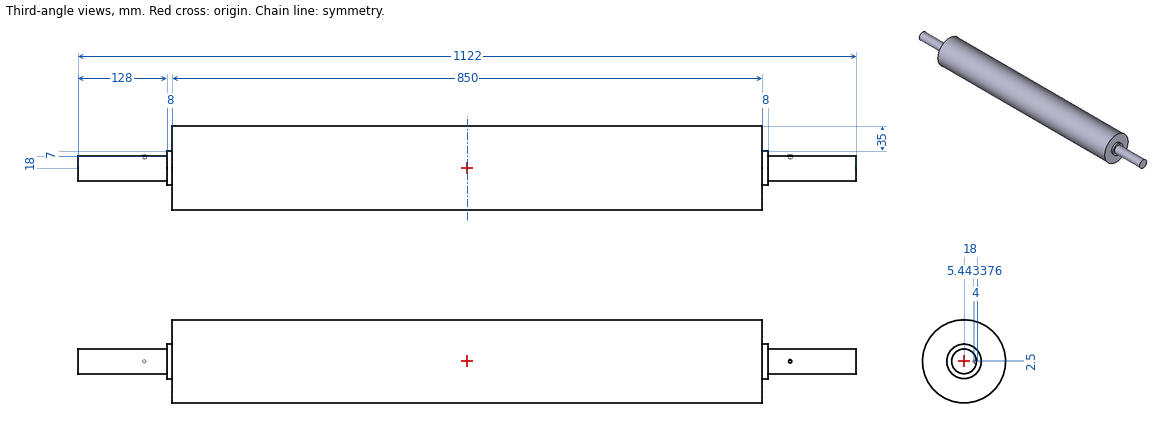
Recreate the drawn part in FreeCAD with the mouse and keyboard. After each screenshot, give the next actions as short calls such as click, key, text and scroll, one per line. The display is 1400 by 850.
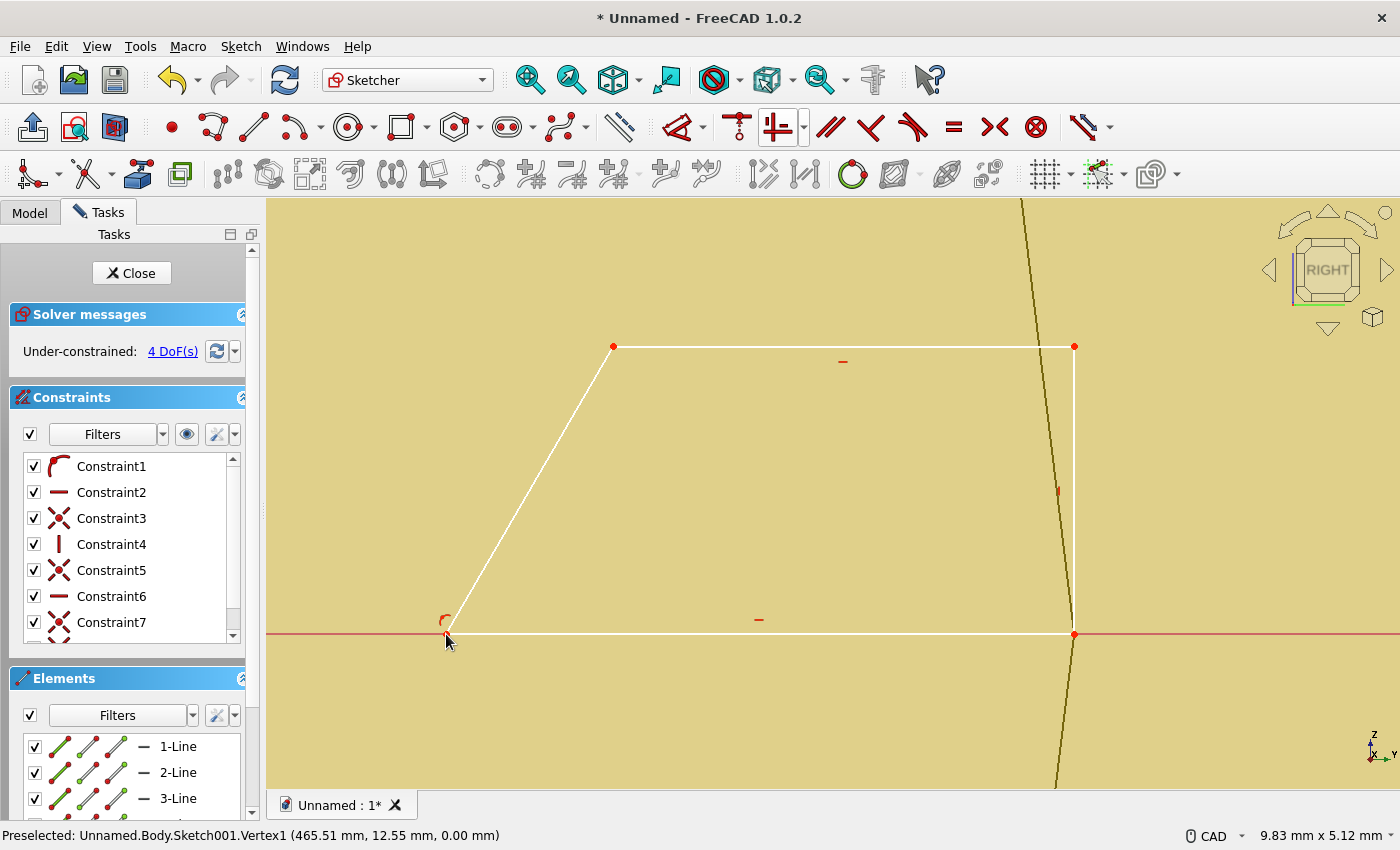
click(676, 128)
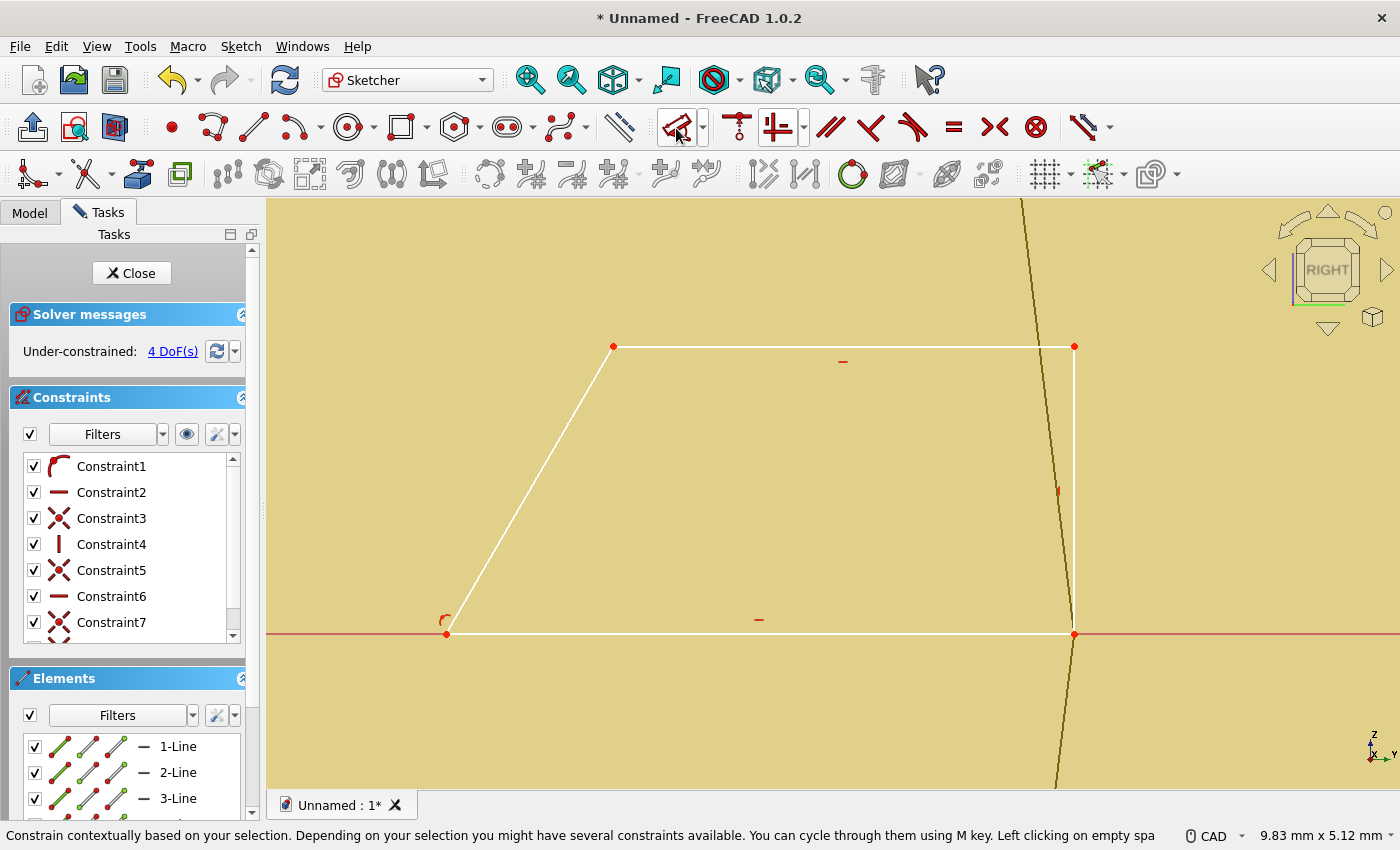
click(936, 347)
click(844, 313)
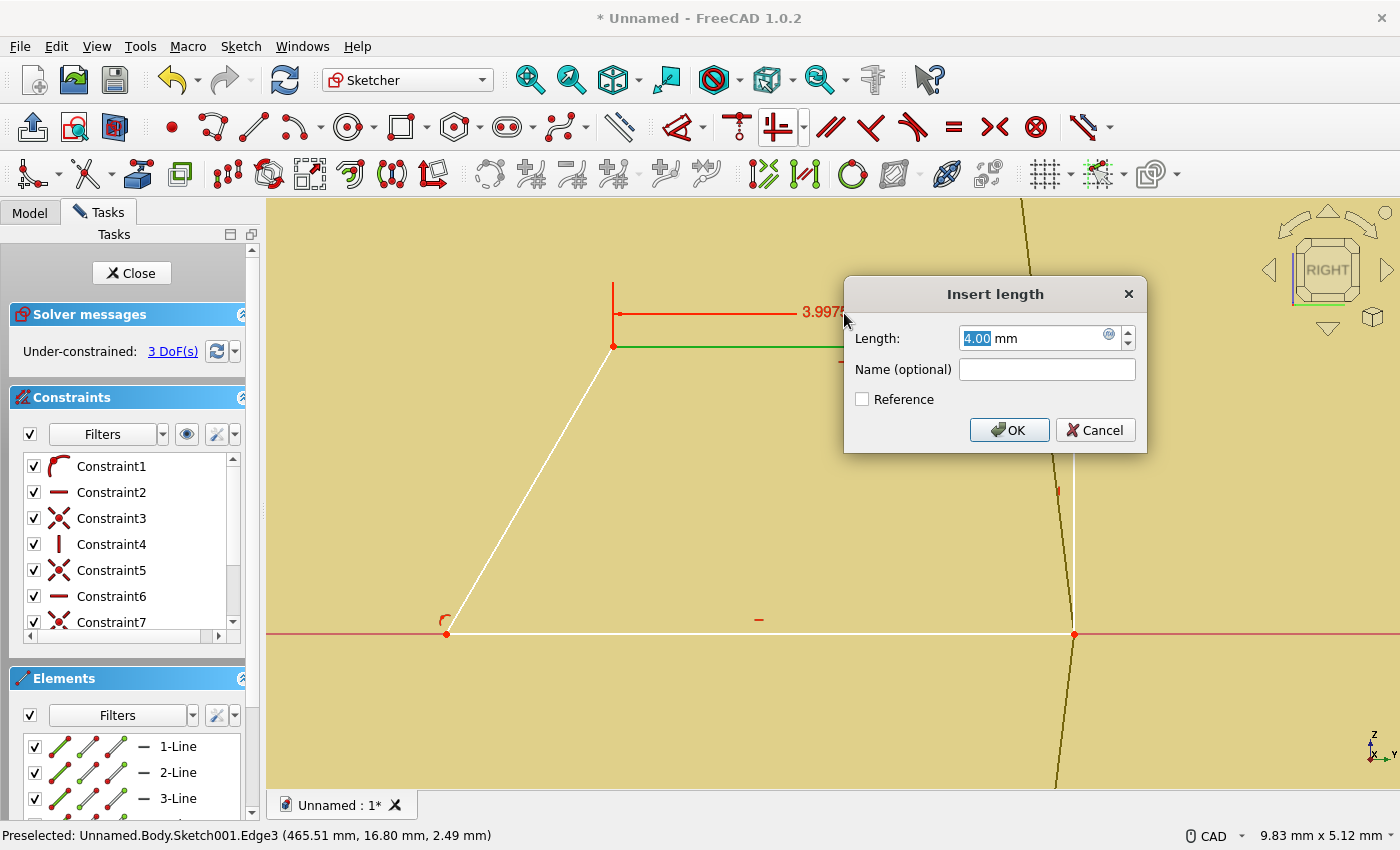
text(4)
key(Return)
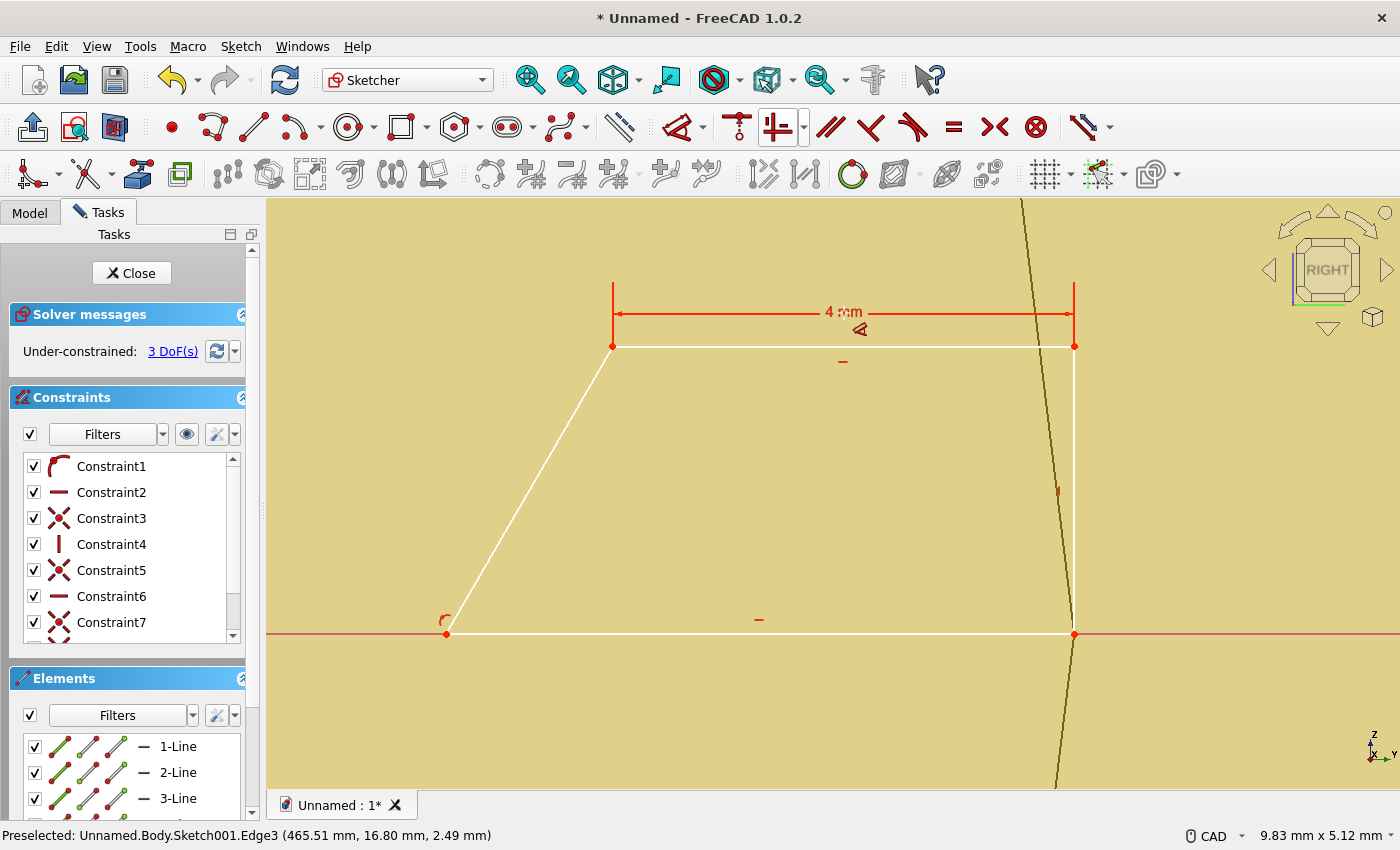
click(1074, 548)
click(1108, 491)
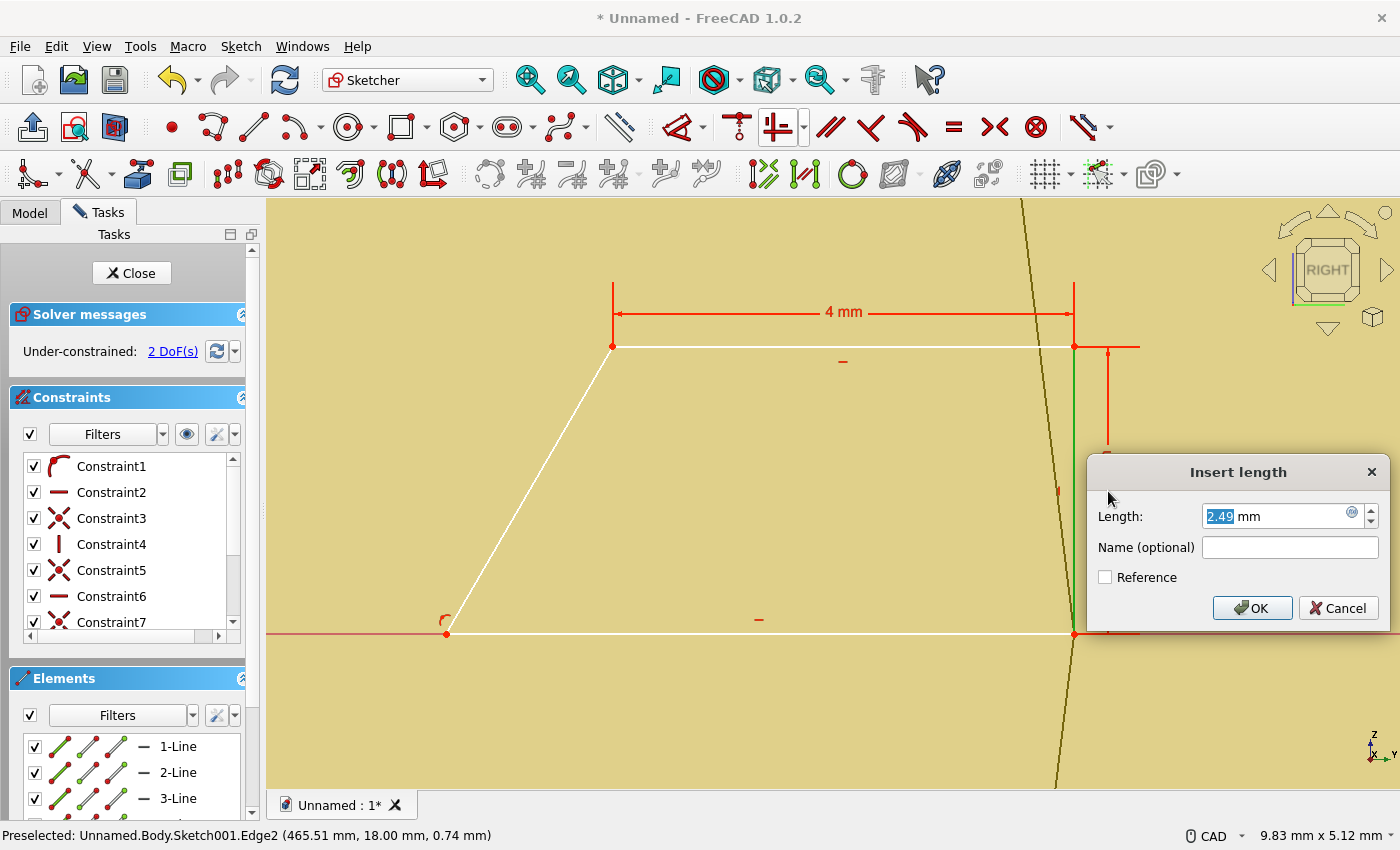
text(2.5)
key(Return)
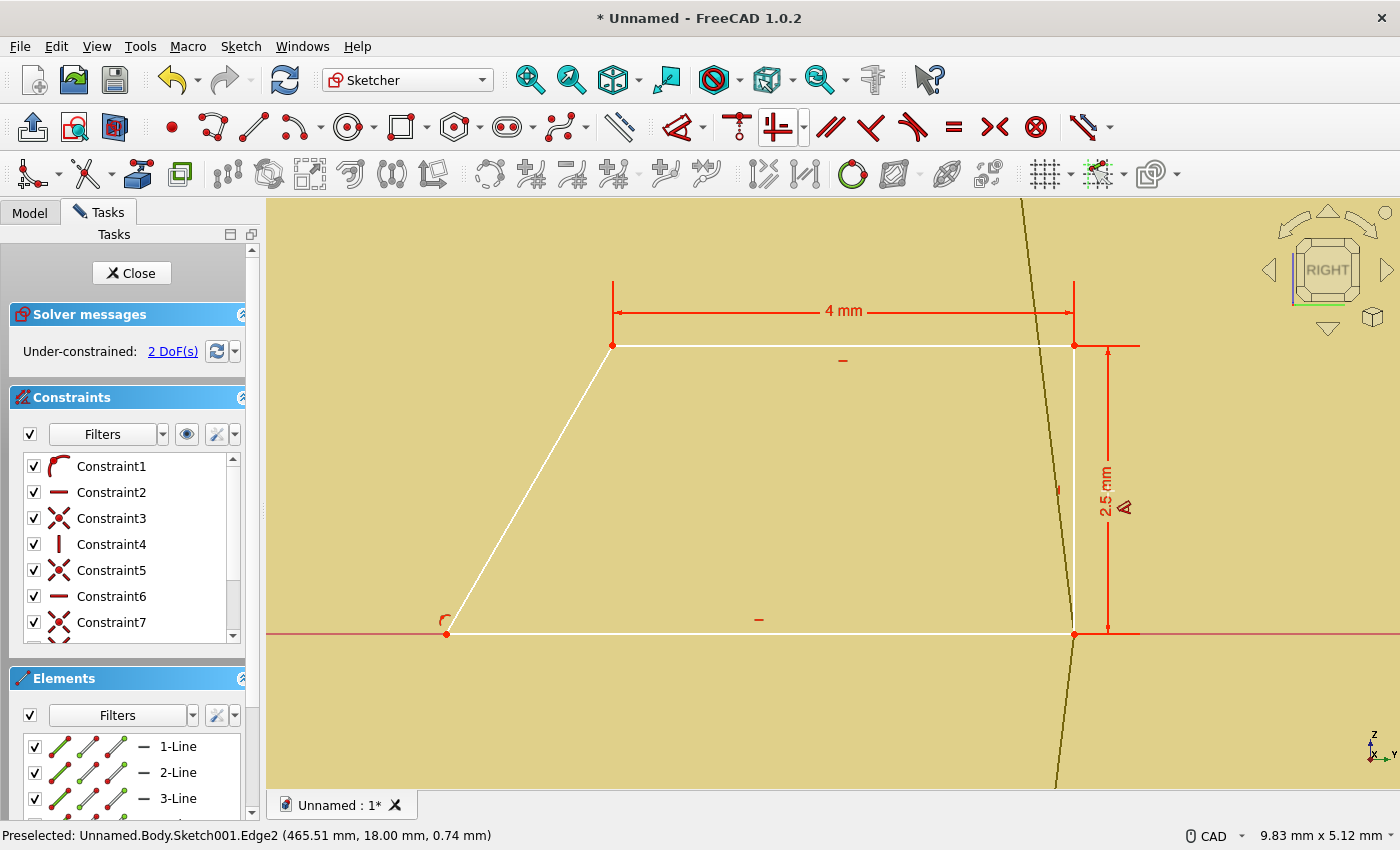
click(1074, 634)
click(684, 668)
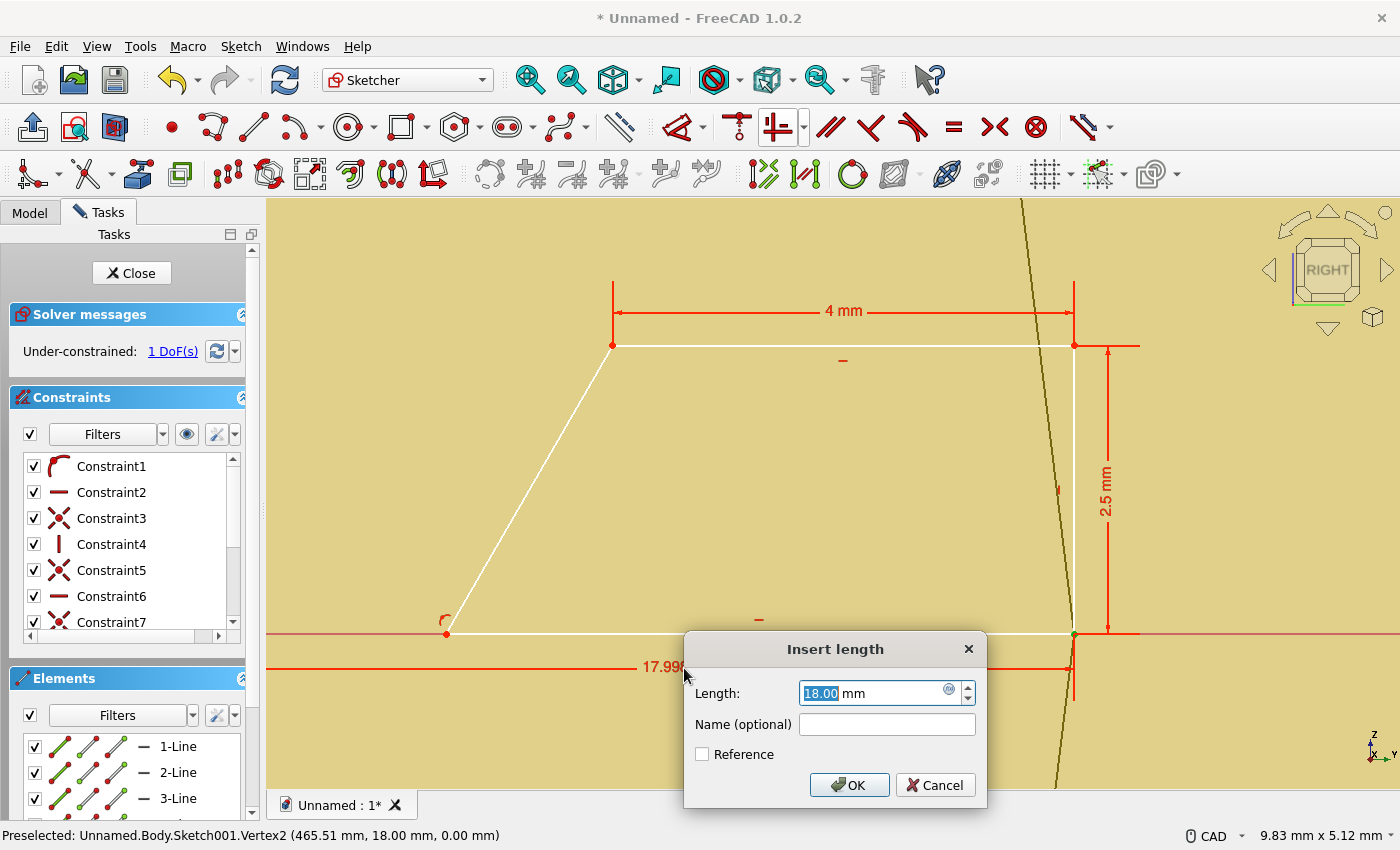
text(18)
key(Return)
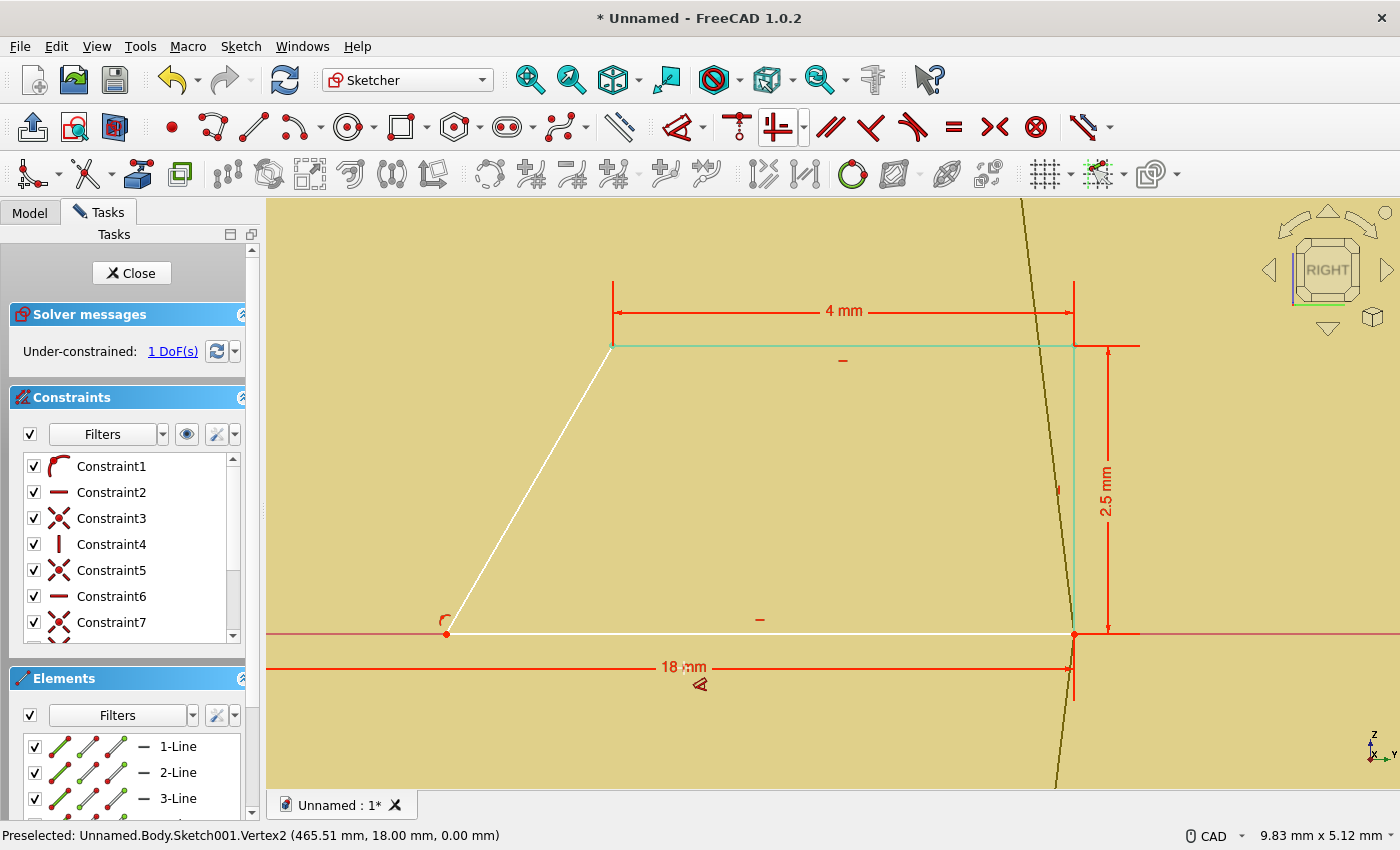
click(634, 634)
click(760, 668)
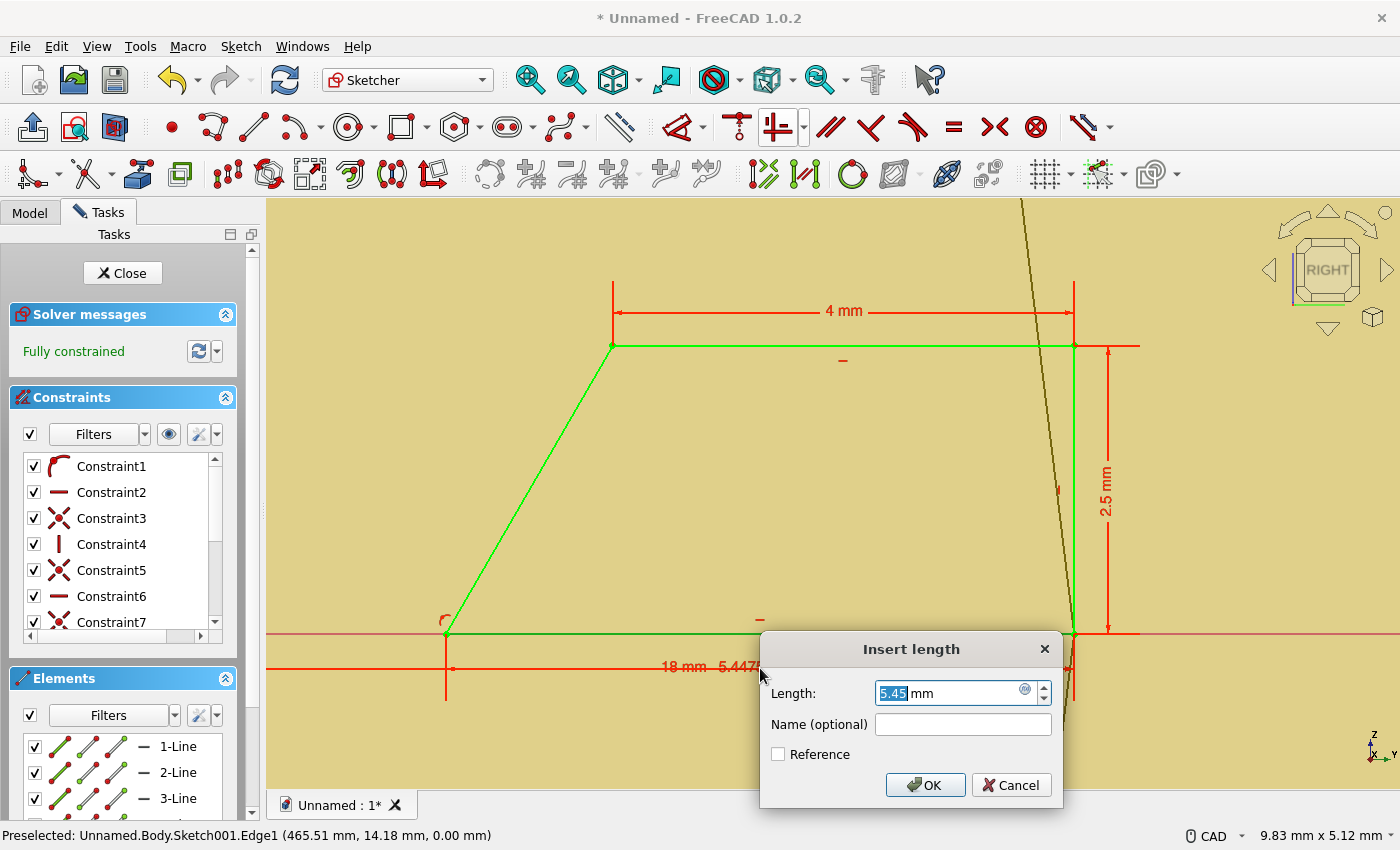
text(5.443376)
key(Return)
key(Escape)